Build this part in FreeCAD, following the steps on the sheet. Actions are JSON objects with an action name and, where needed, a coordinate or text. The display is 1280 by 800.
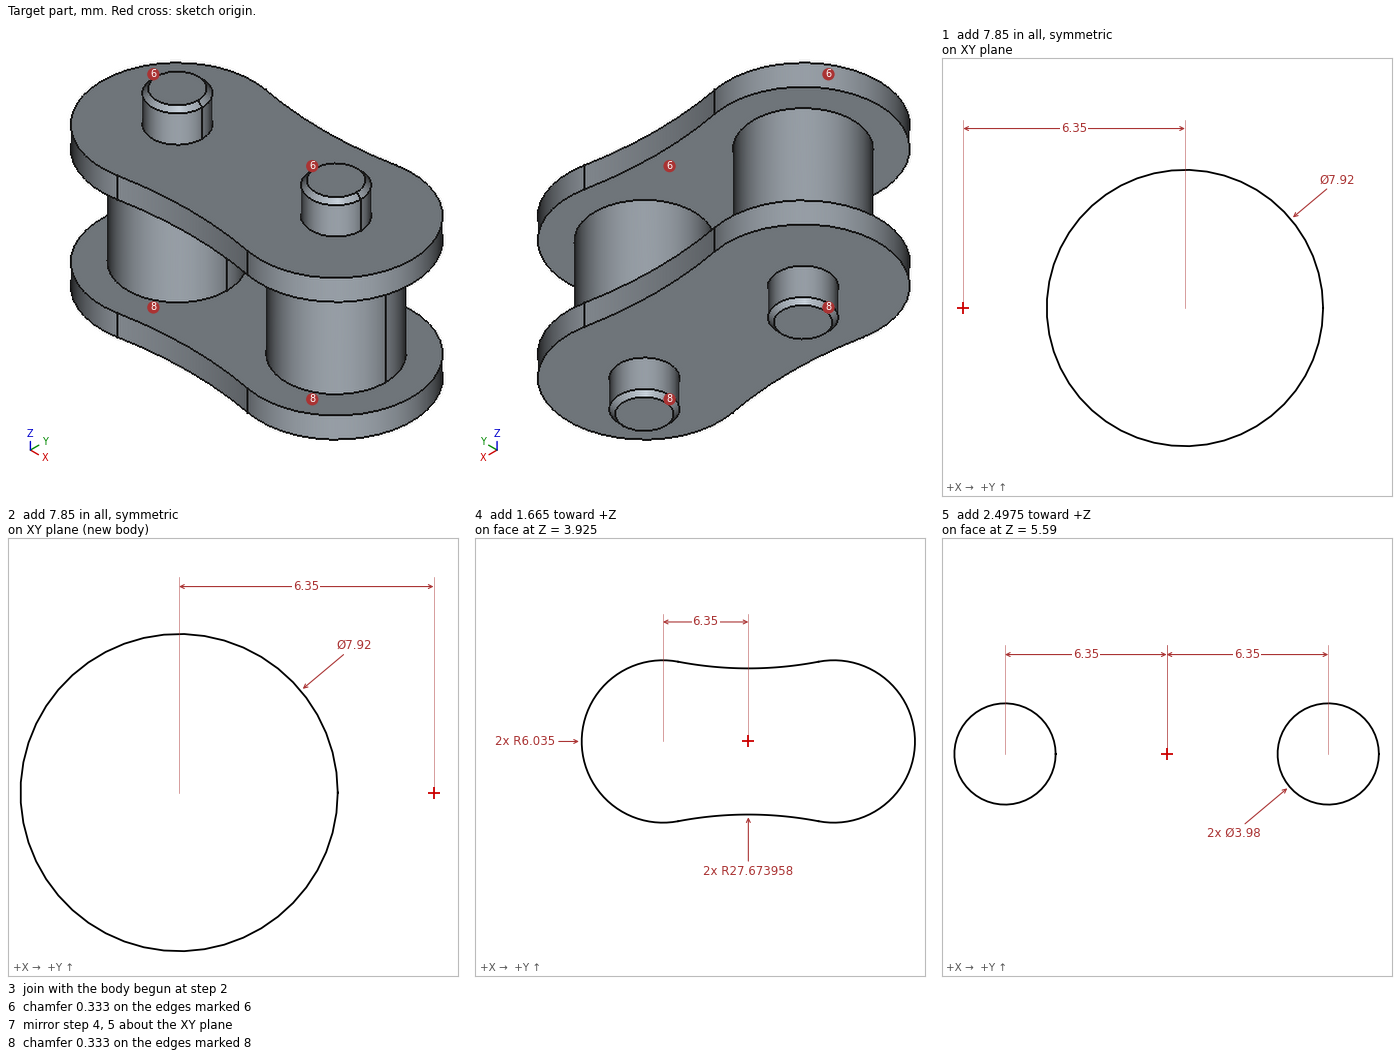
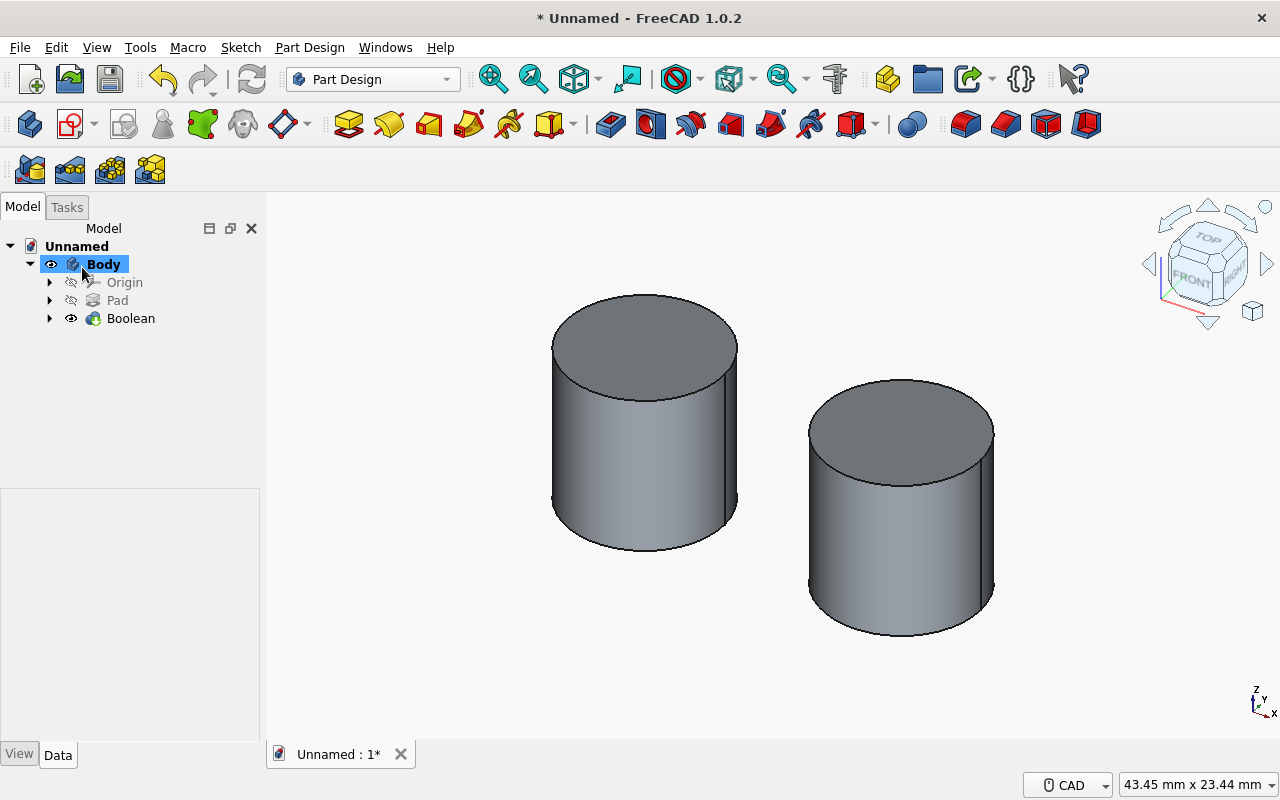
{"action": "left_click", "coordinate": [645, 347]}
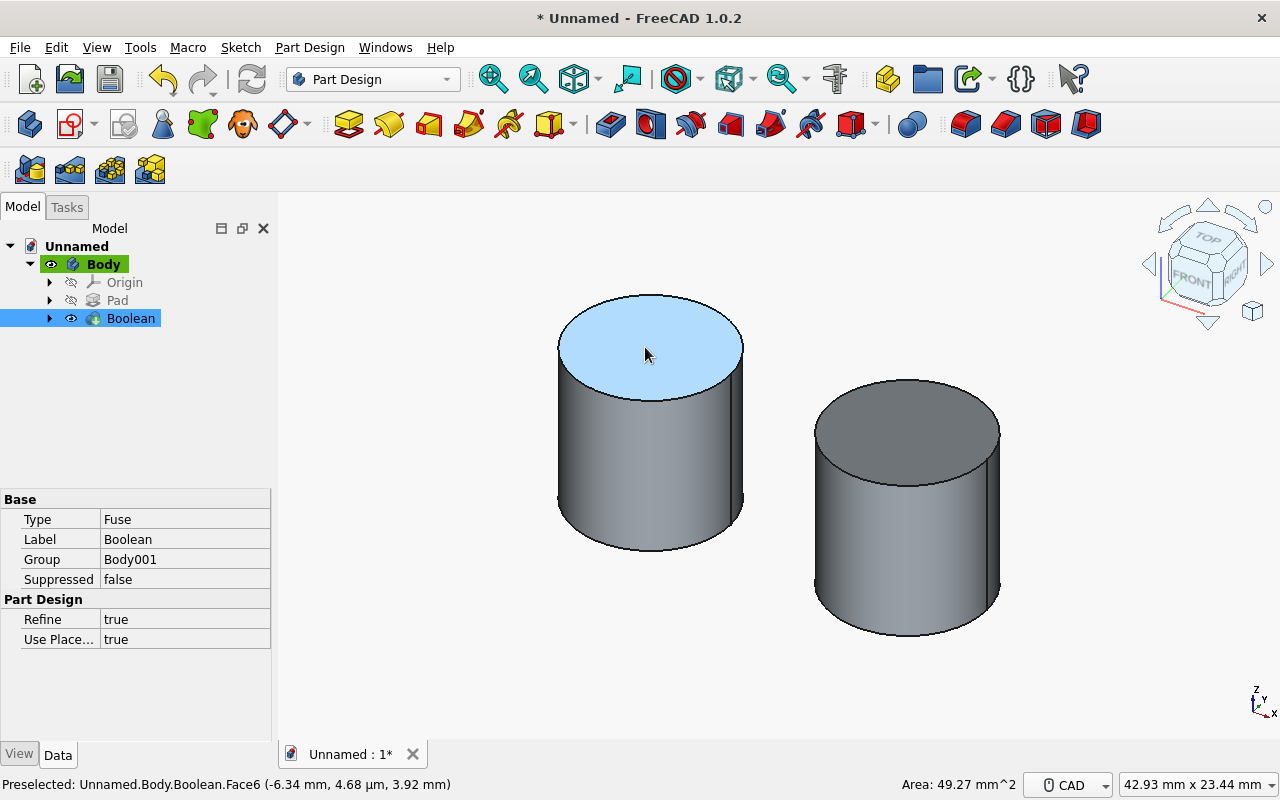
{"action": "left_click", "coordinate": [70, 124]}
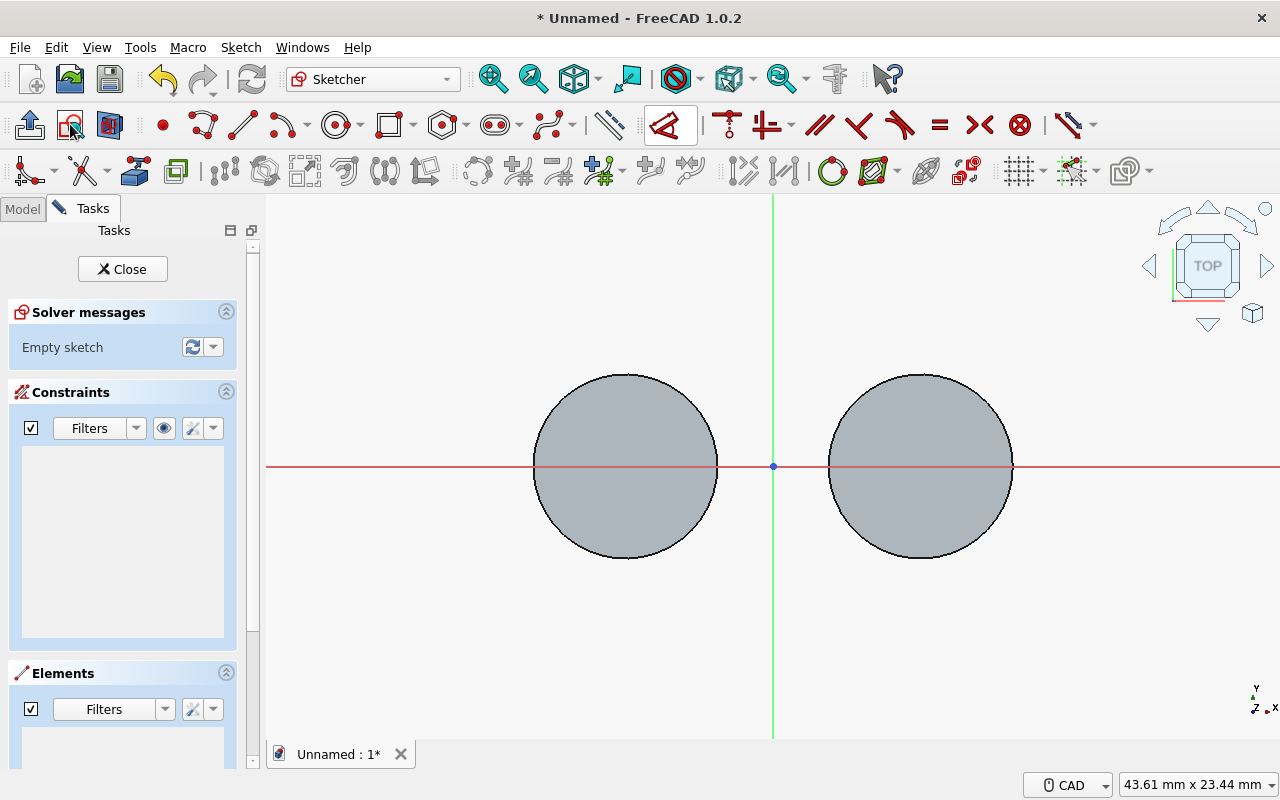
{"action": "left_click", "coordinate": [310, 126]}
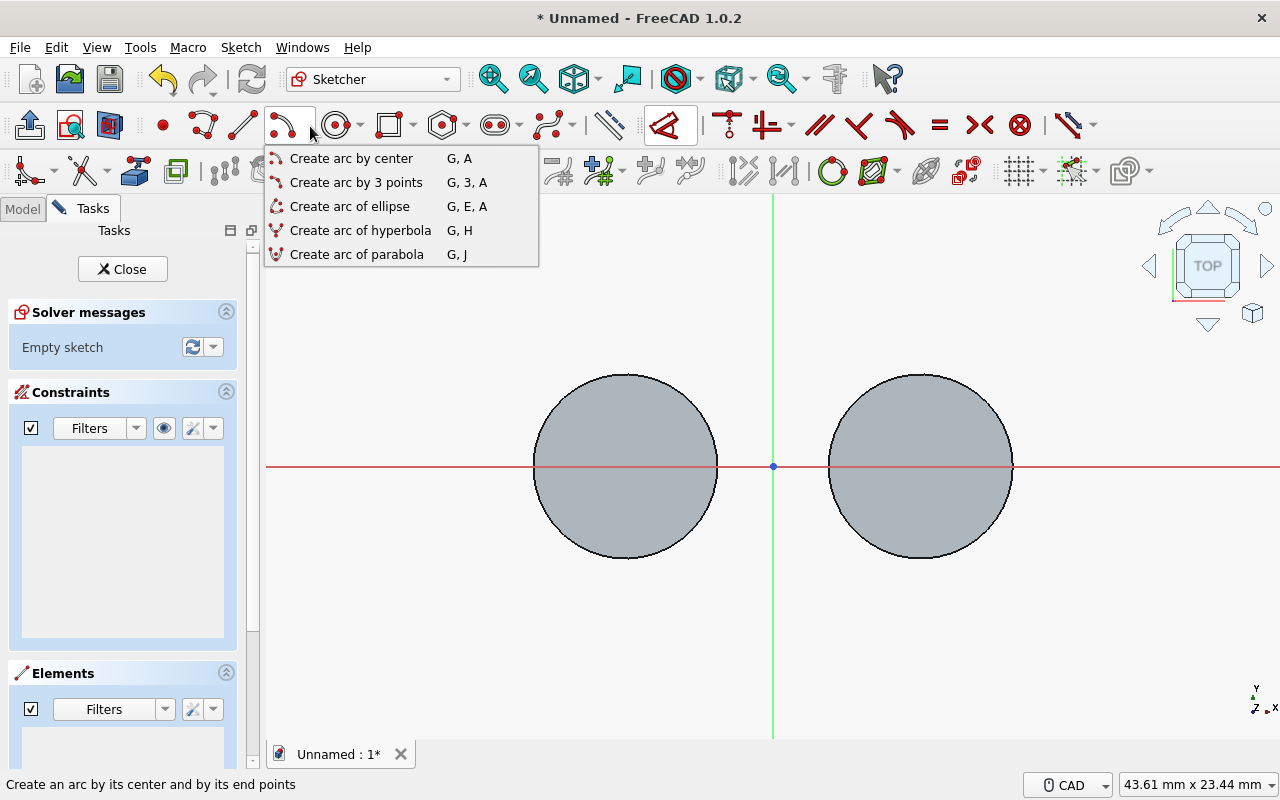
{"action": "left_click", "coordinate": [402, 182]}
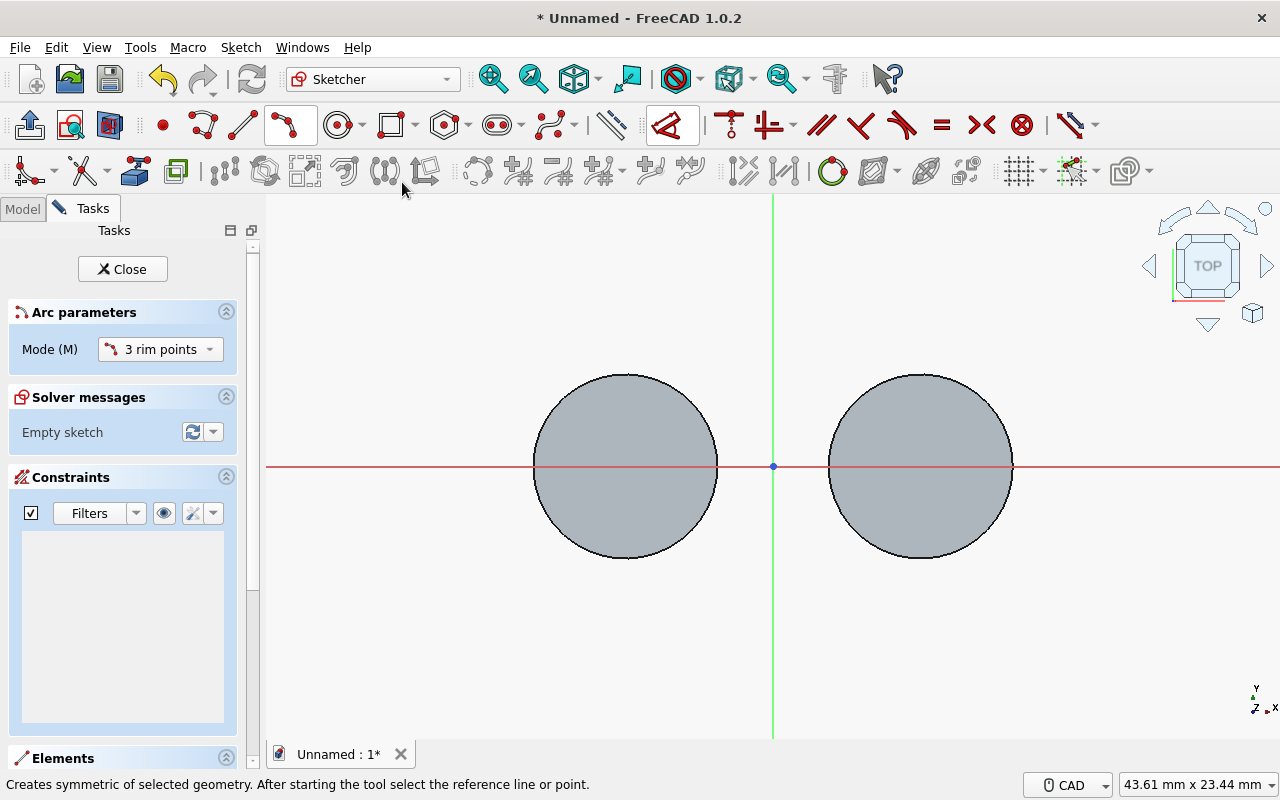
{"action": "left_click", "coordinate": [652, 329]}
{"action": "left_click", "coordinate": [652, 604]}
{"action": "left_click", "coordinate": [494, 418]}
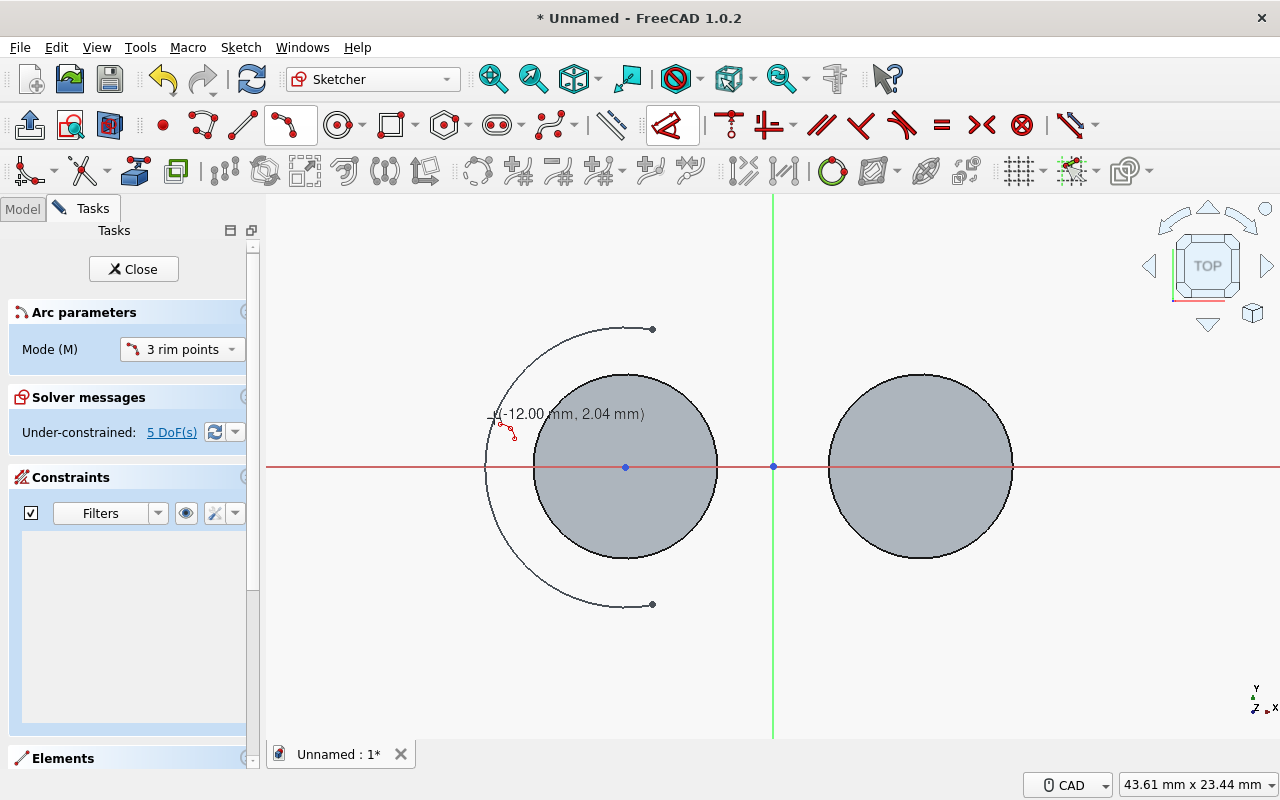
{"action": "left_click", "coordinate": [652, 605]}
{"action": "left_click", "coordinate": [894, 604]}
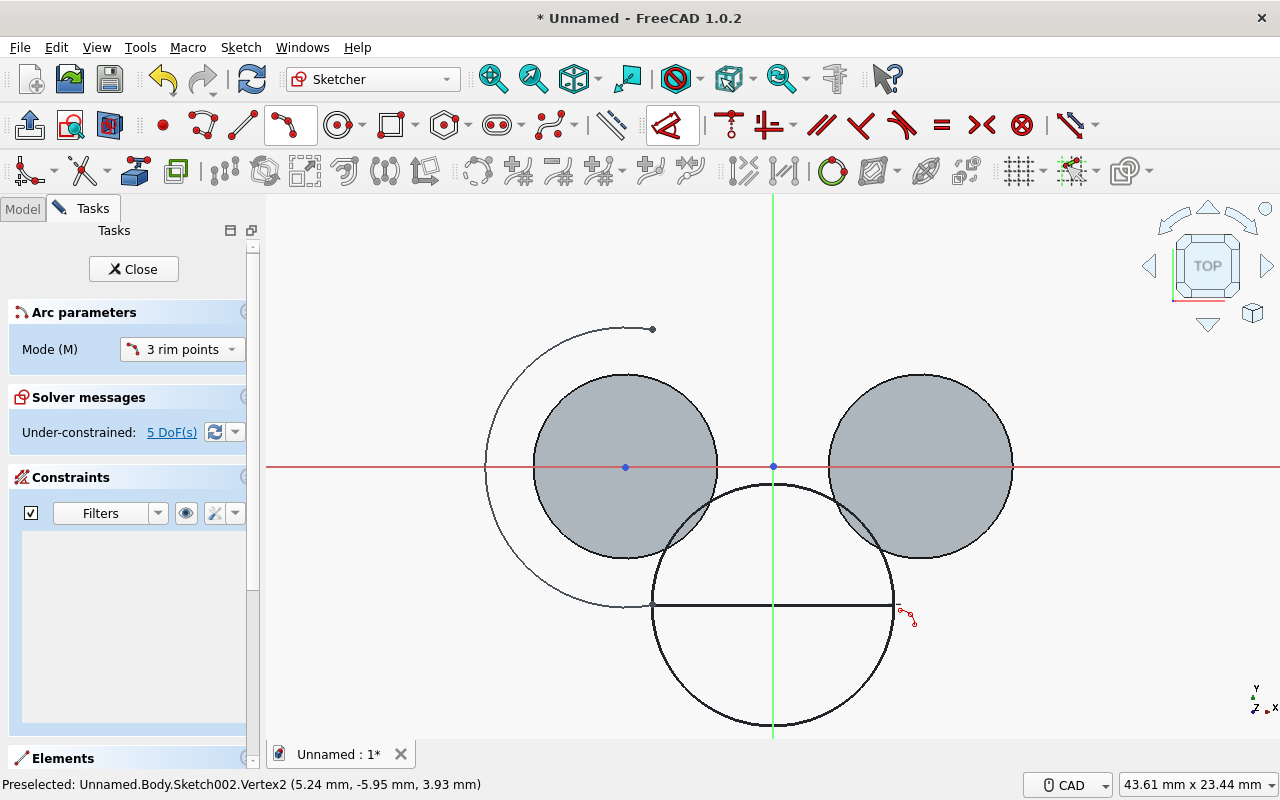
{"action": "scroll", "coordinate": [797, 593], "scroll_direction": "up", "scroll_amount": 2}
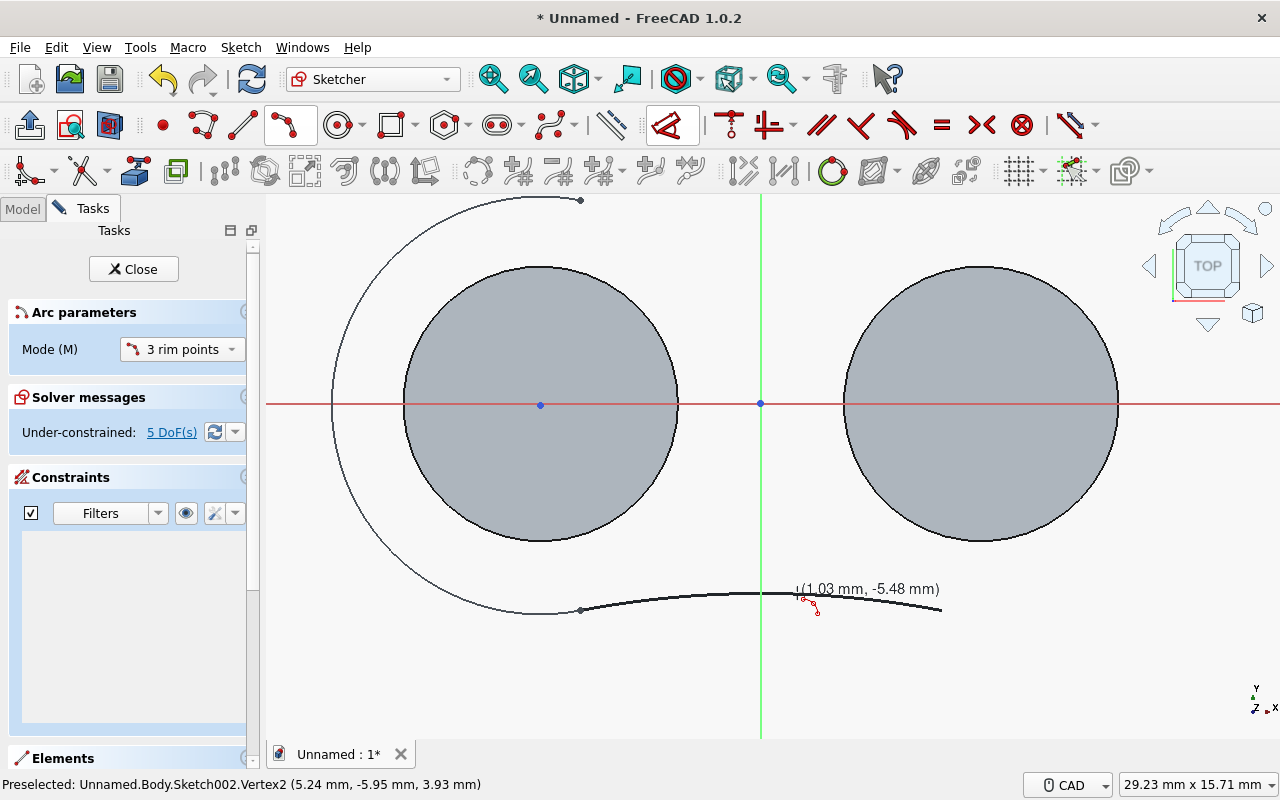
{"action": "left_click", "coordinate": [797, 593]}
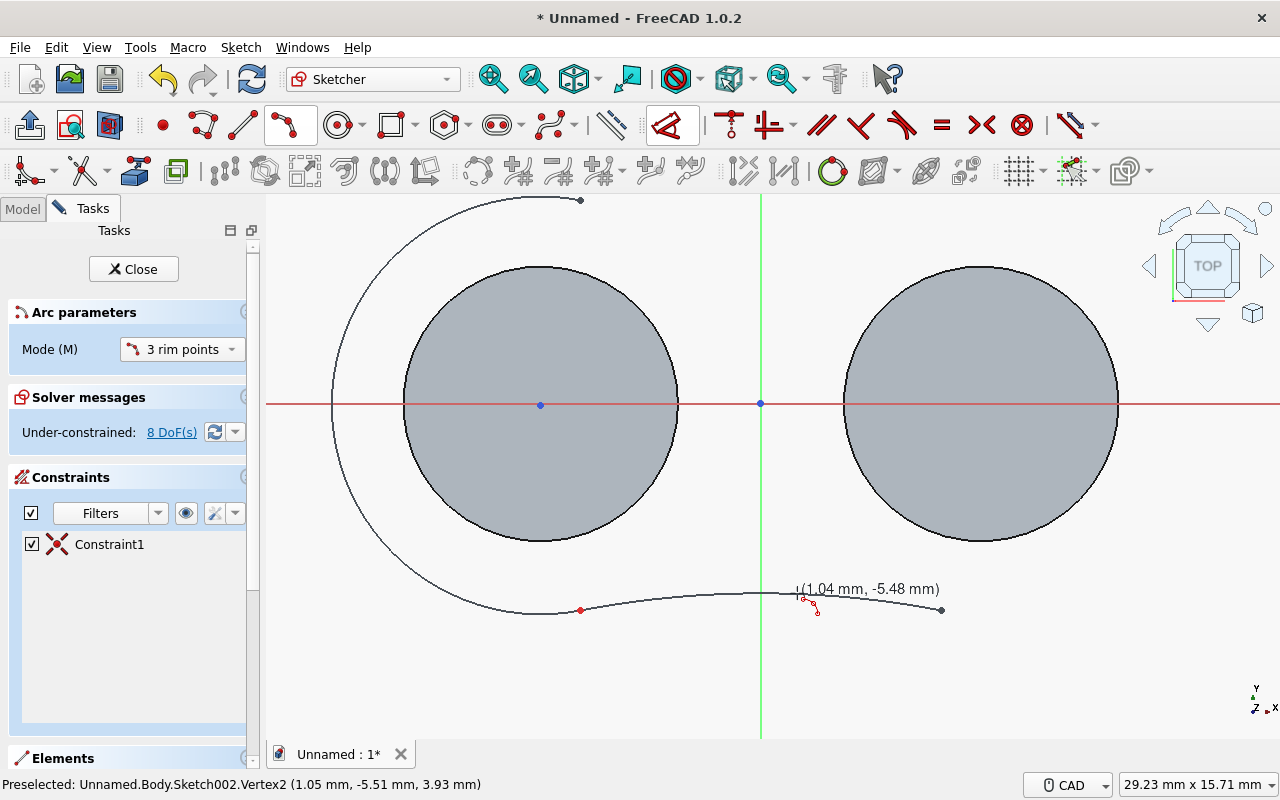
{"action": "left_click", "coordinate": [941, 611]}